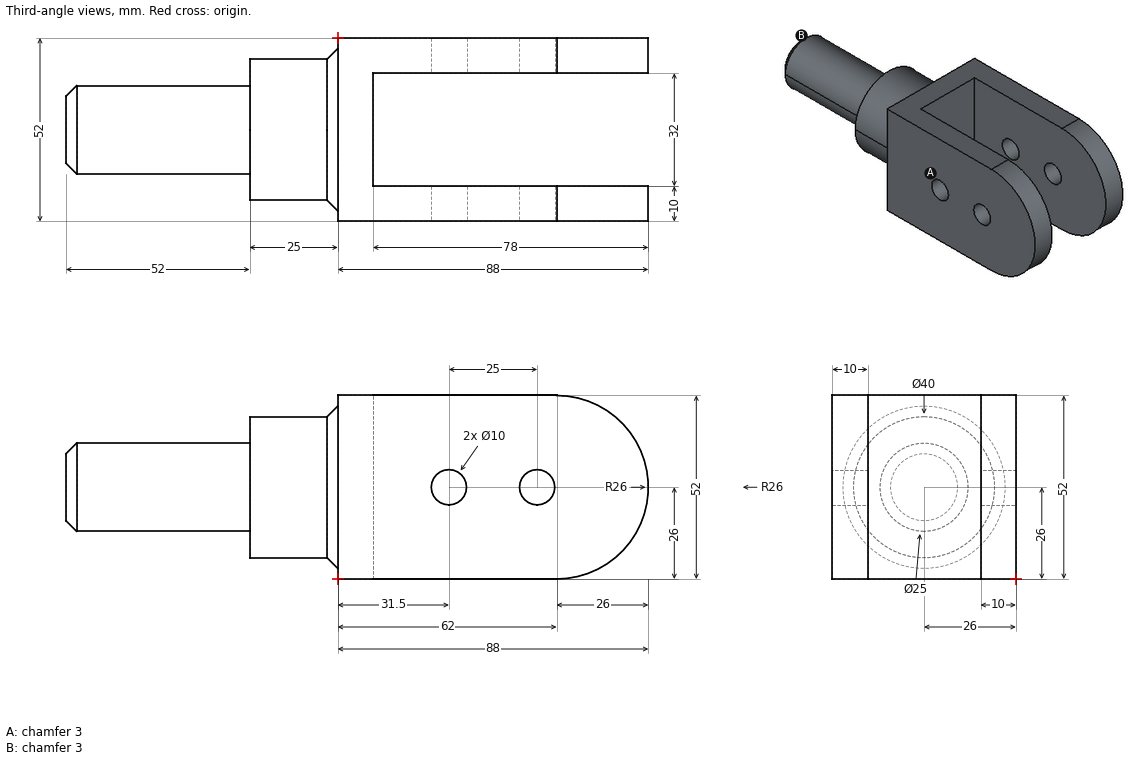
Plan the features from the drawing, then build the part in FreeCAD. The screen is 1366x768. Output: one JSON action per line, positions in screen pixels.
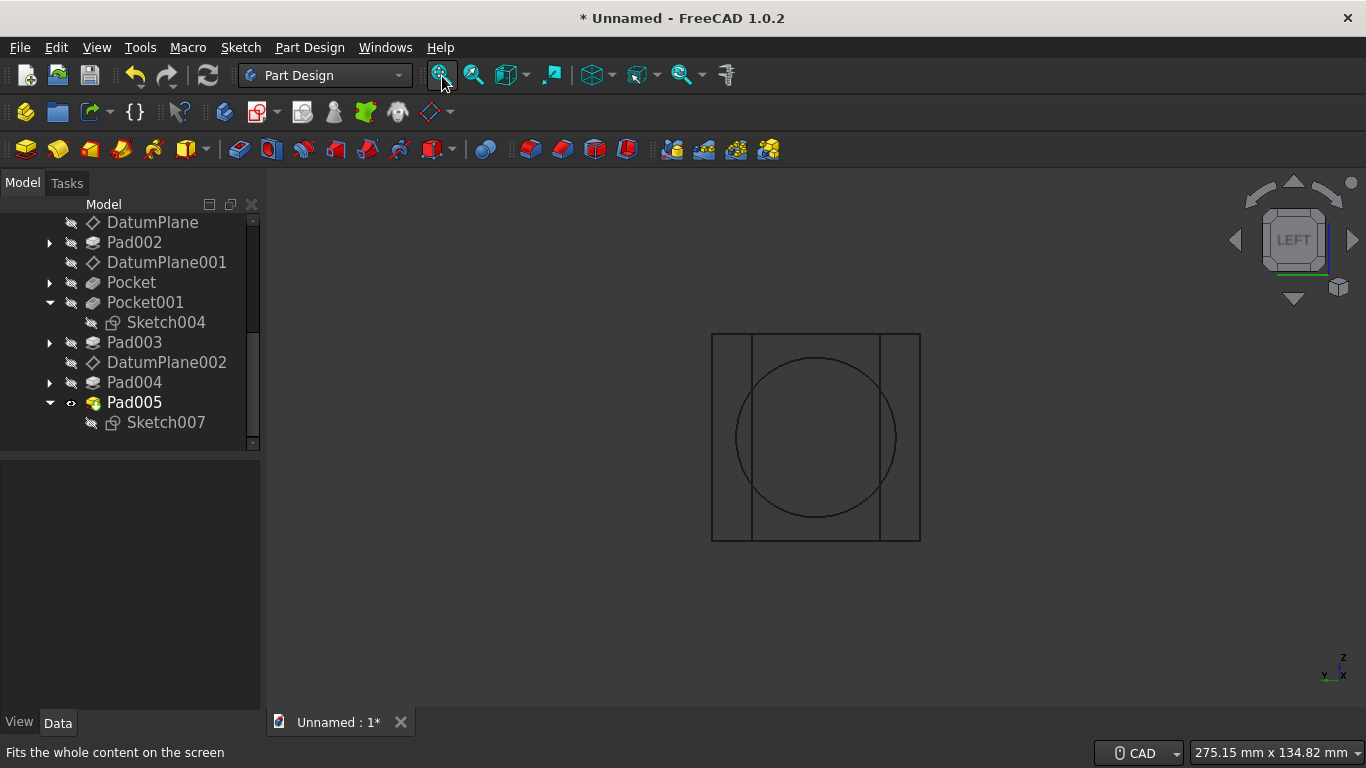
{"action": "key", "text": "0"}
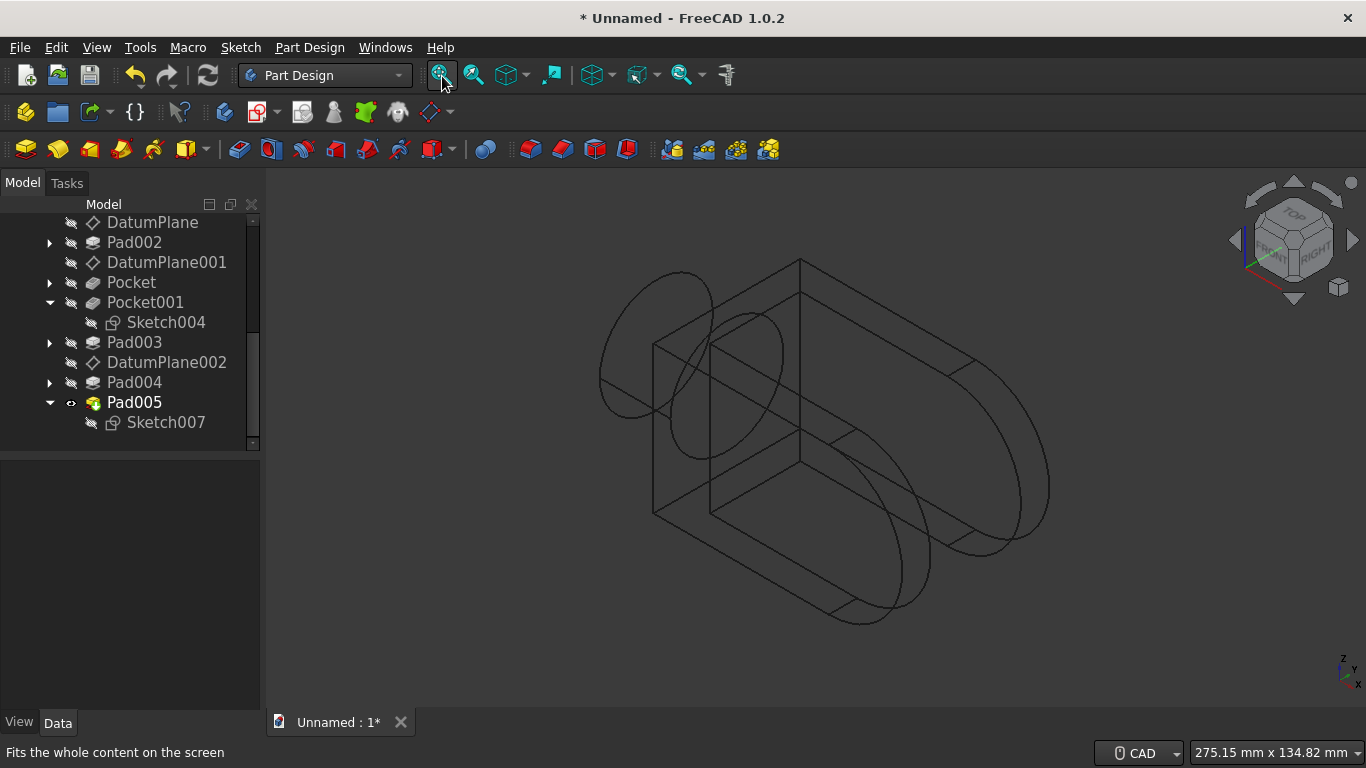
{"action": "left_click", "coordinate": [783, 352]}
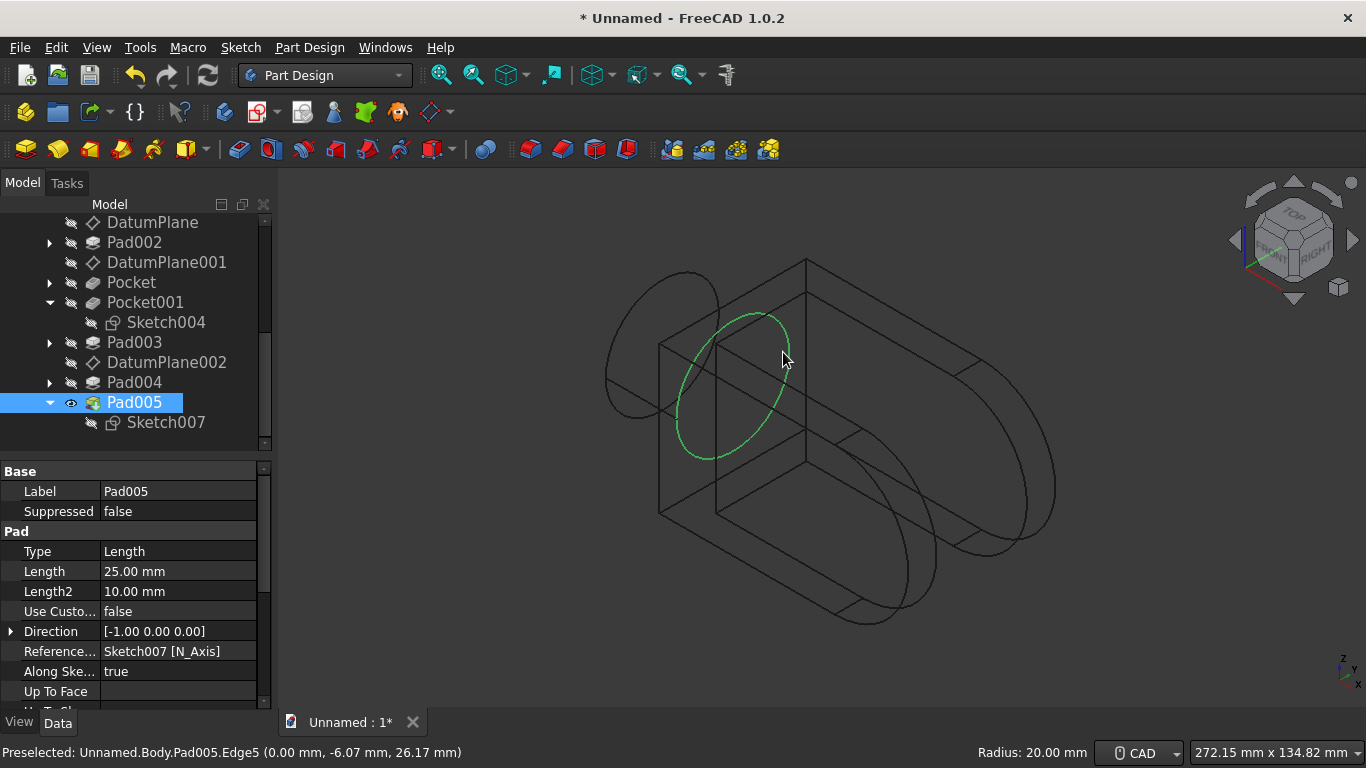
{"action": "key", "text": "v 1"}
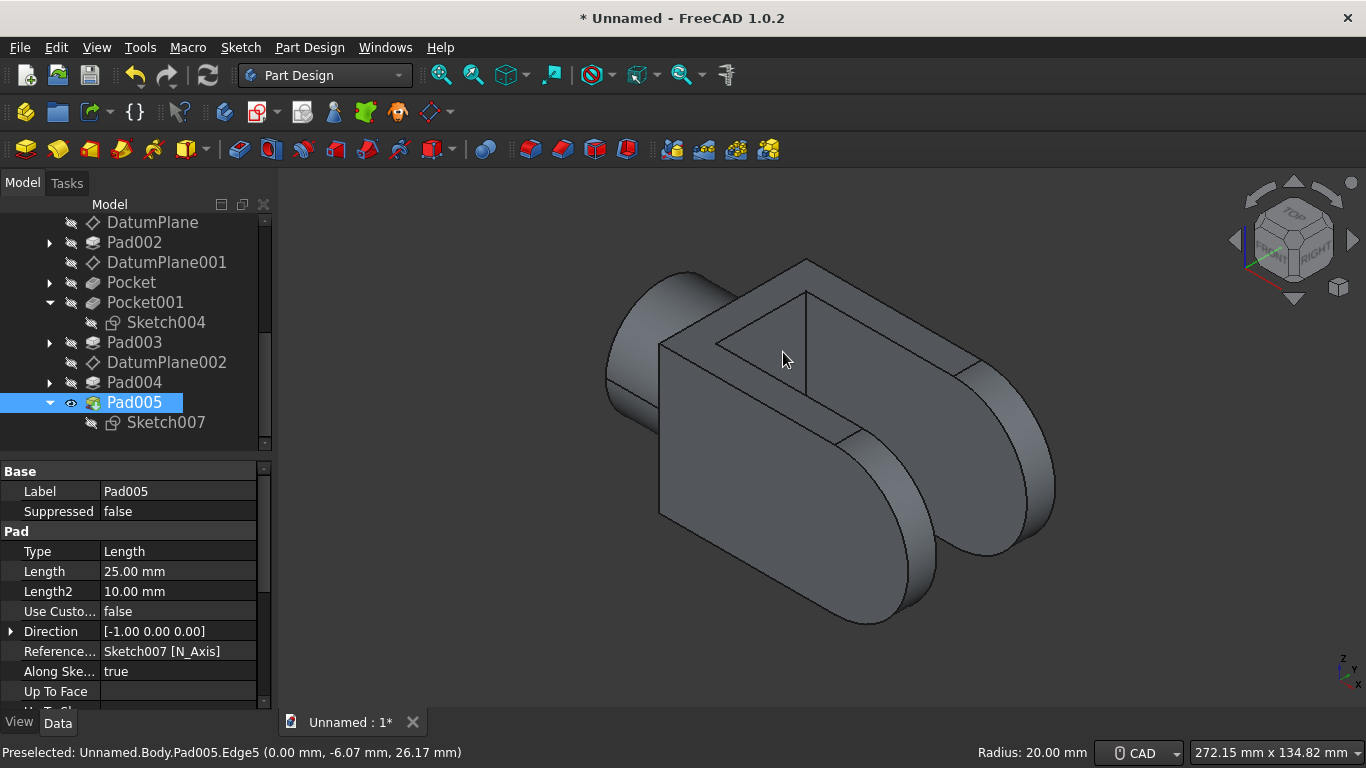
{"action": "left_click", "coordinate": [564, 150]}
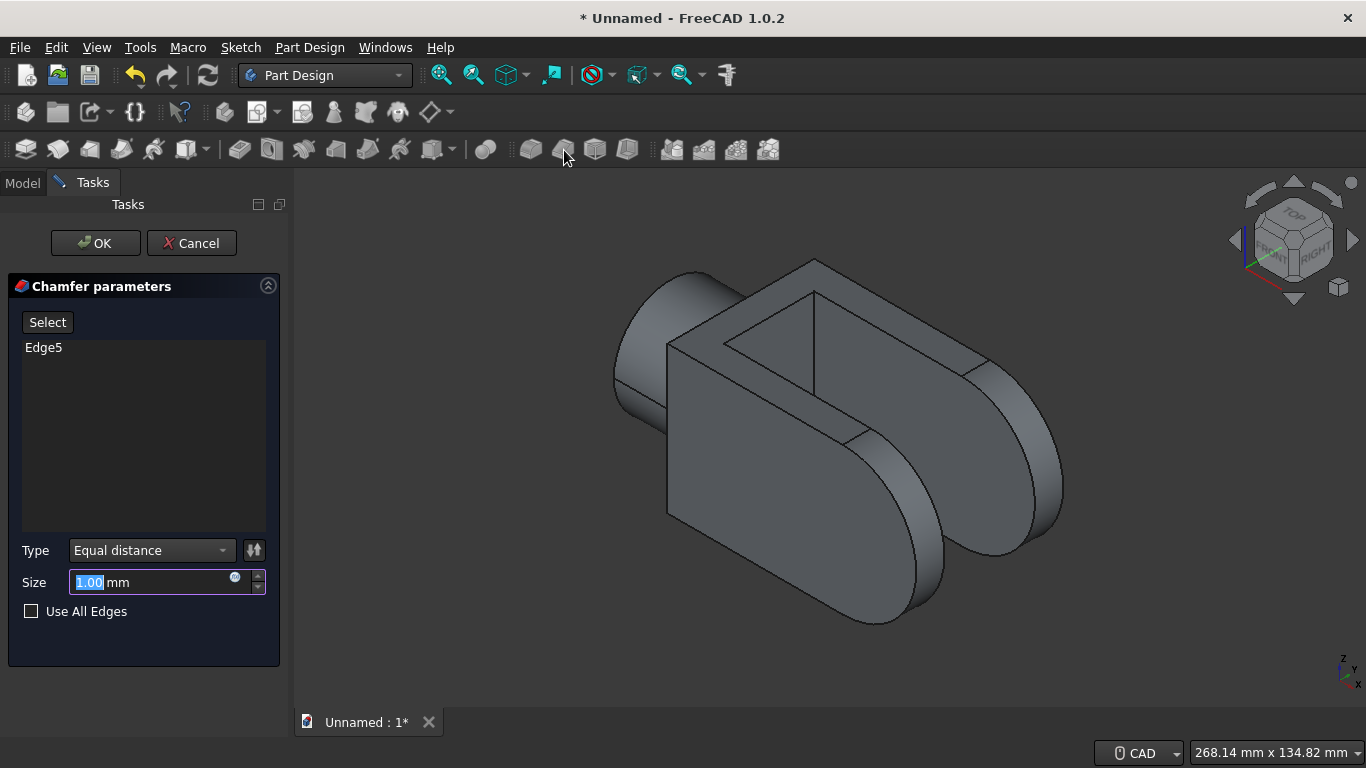
{"action": "type", "text": "3"}
{"action": "key", "text": "Tab"}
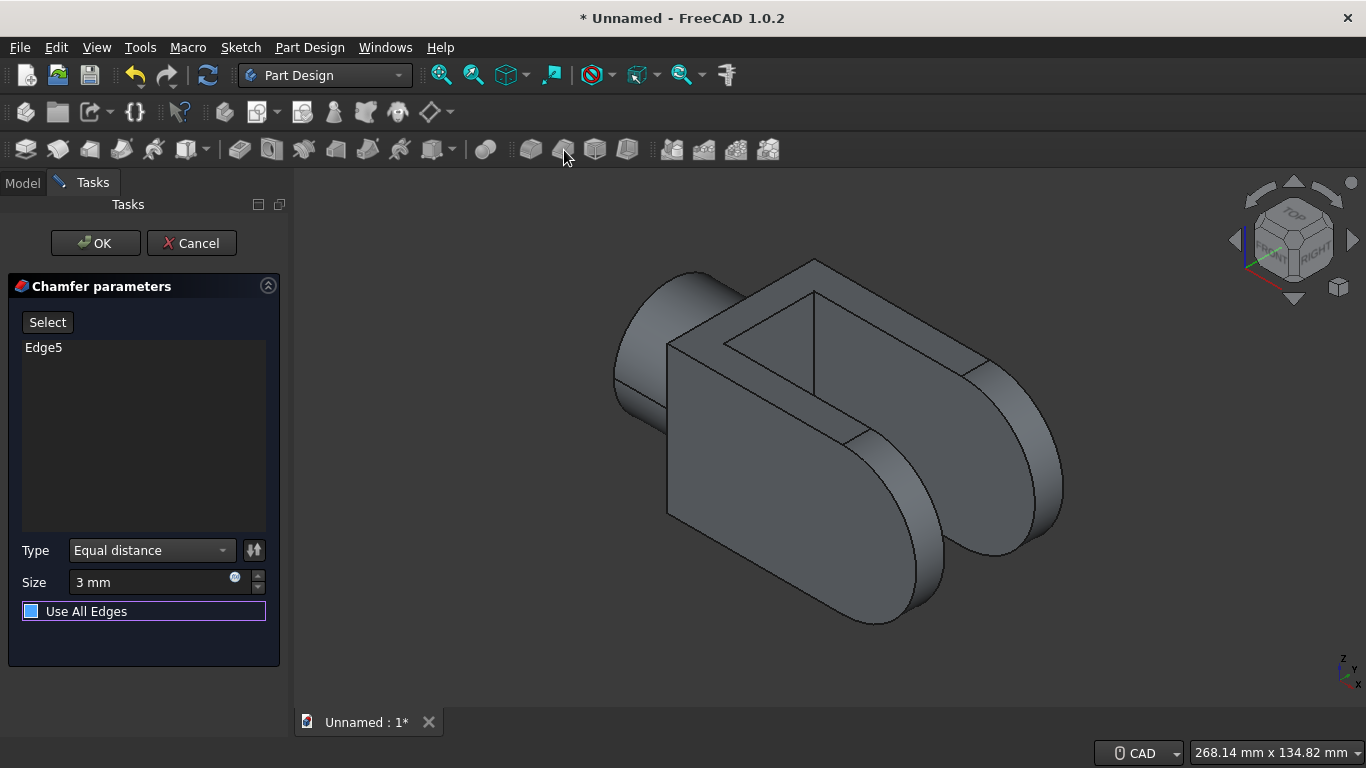
{"action": "left_click", "coordinate": [96, 243]}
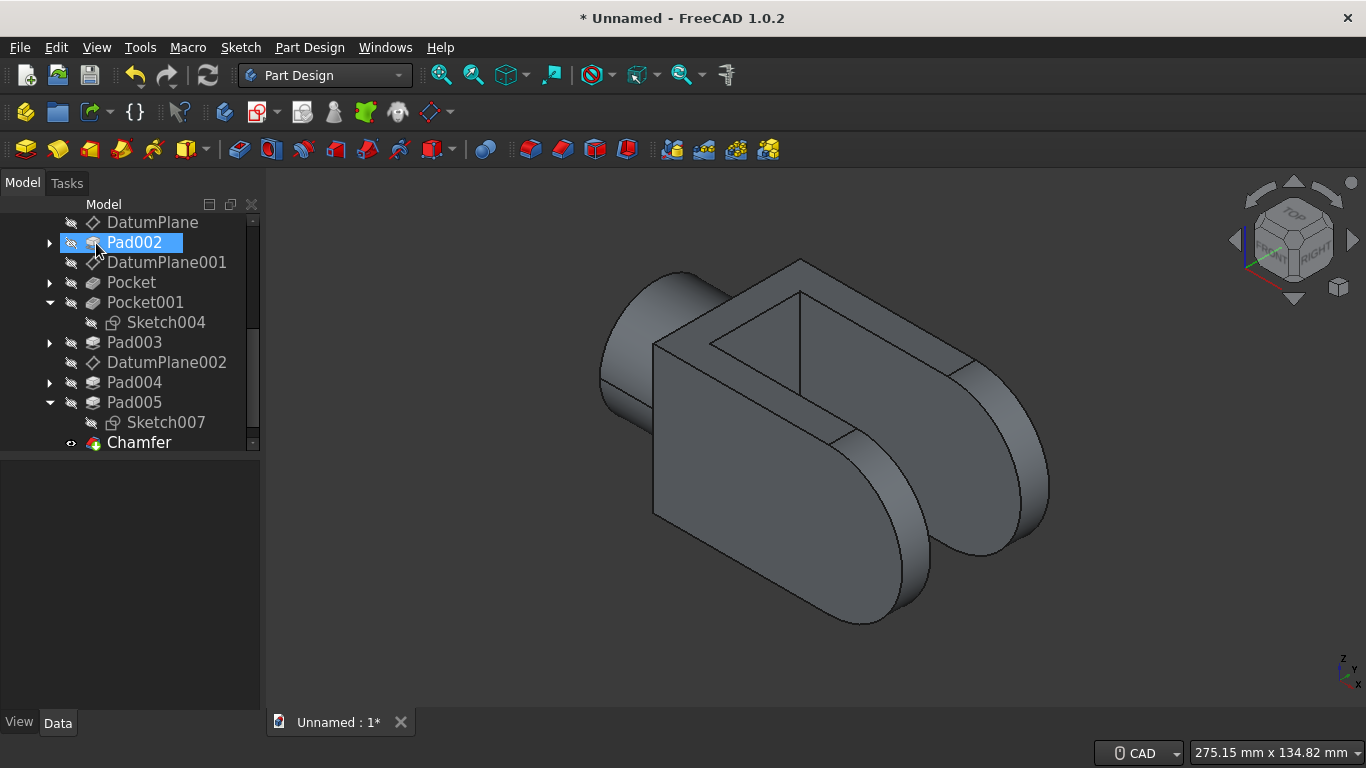
{"action": "key", "text": "6"}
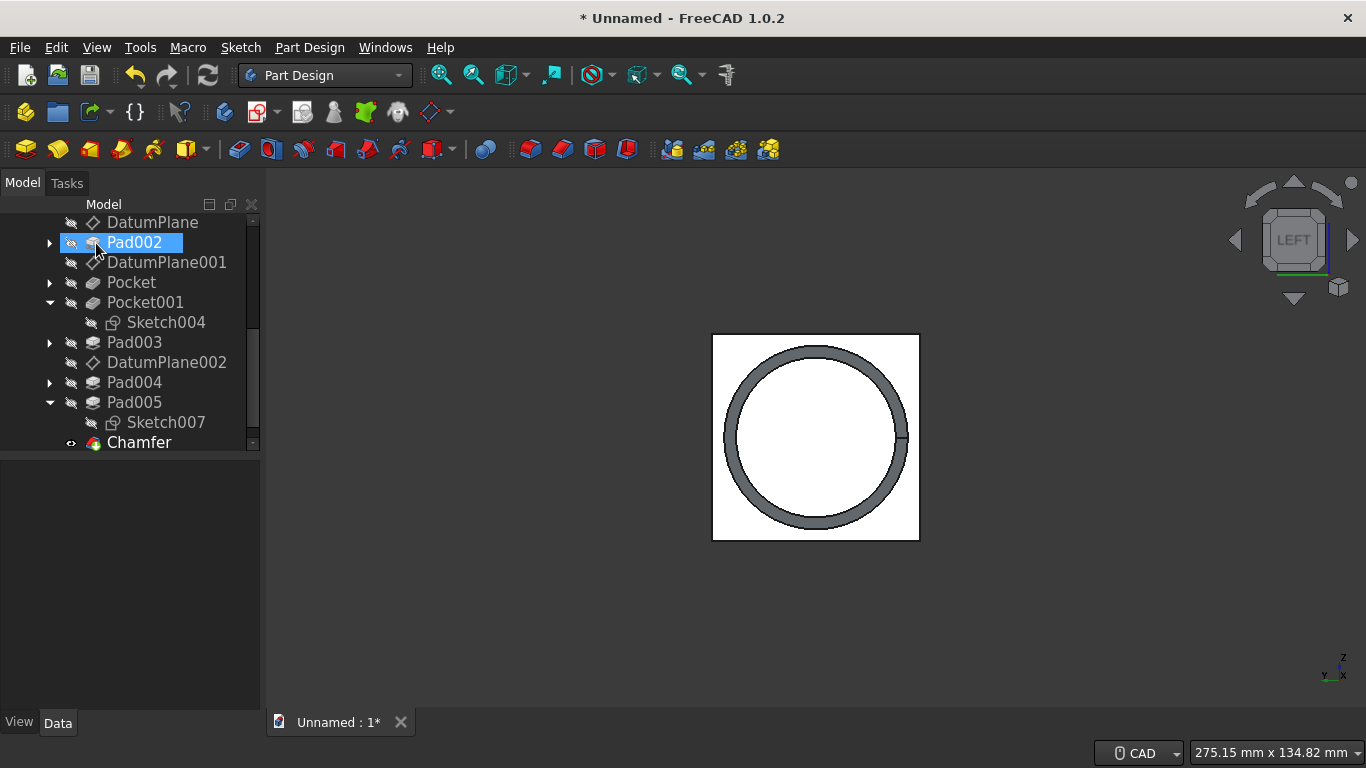
{"action": "left_click", "coordinate": [442, 76]}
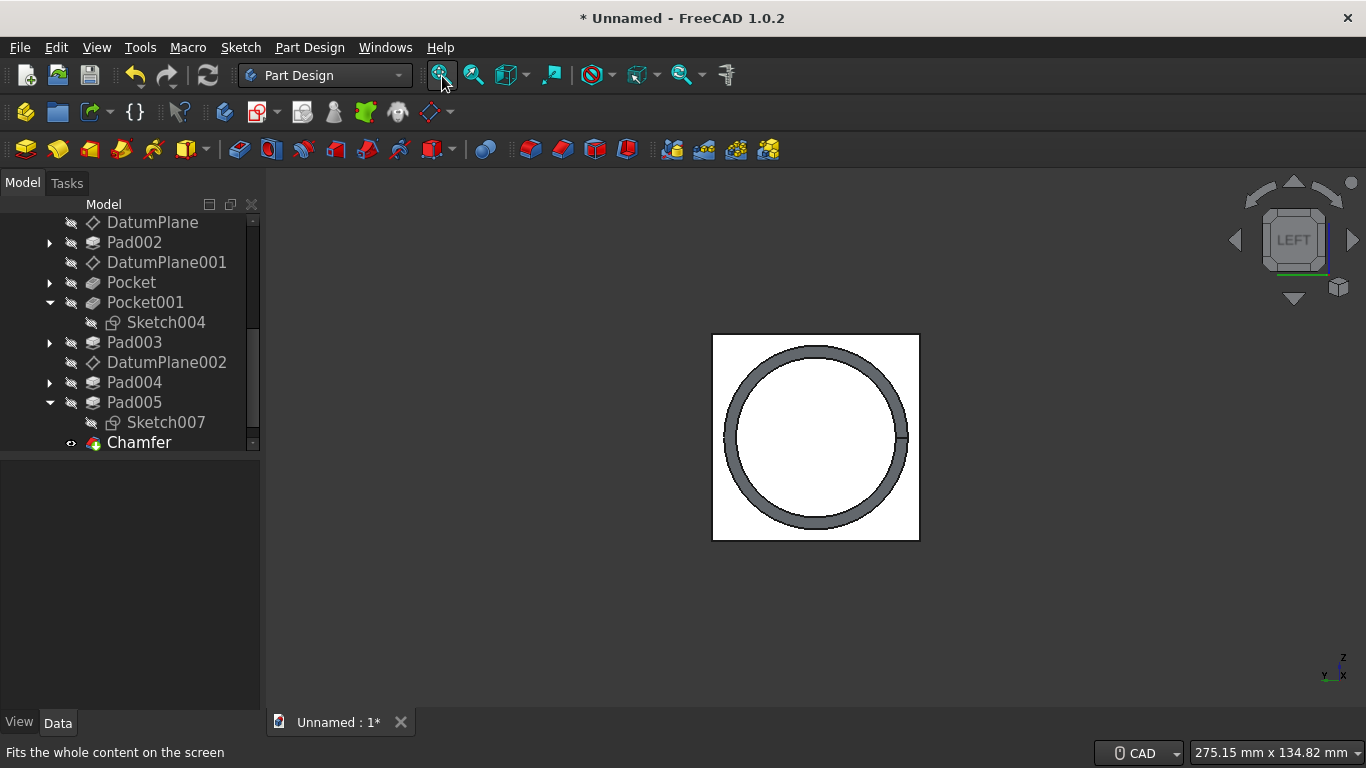
{"action": "left_click", "coordinate": [816, 436]}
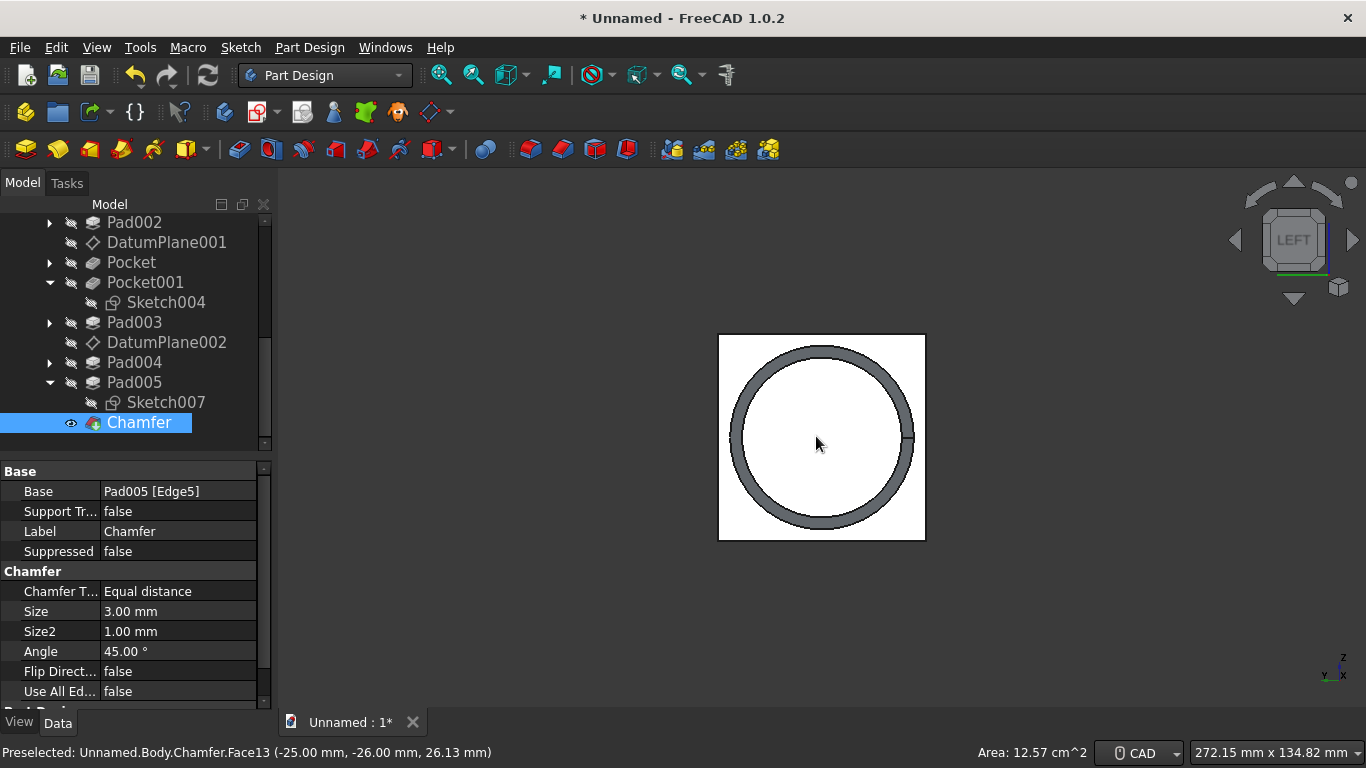
{"action": "left_click", "coordinate": [258, 112]}